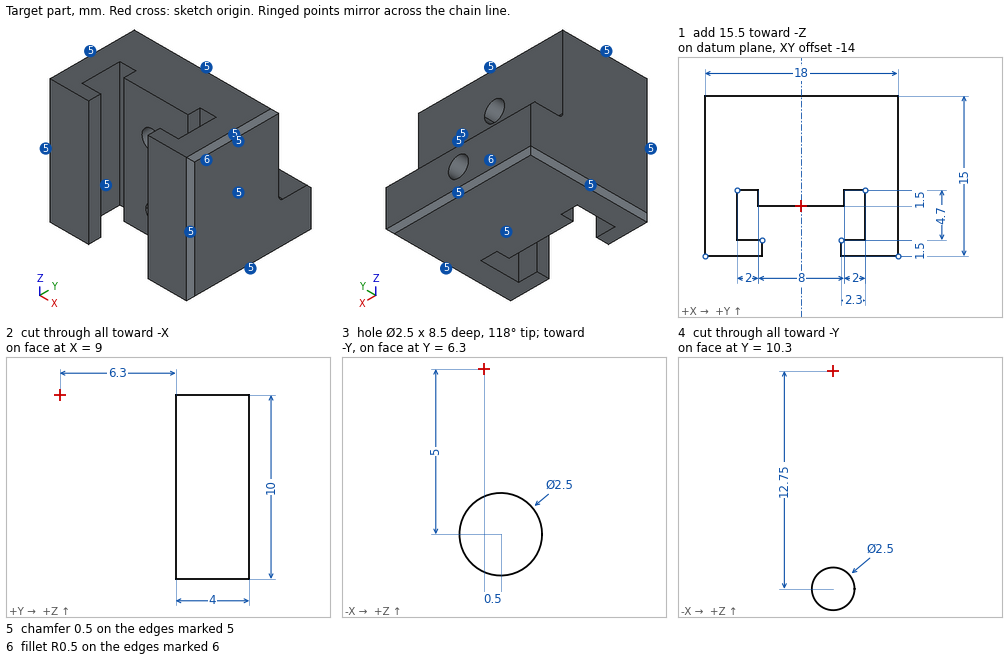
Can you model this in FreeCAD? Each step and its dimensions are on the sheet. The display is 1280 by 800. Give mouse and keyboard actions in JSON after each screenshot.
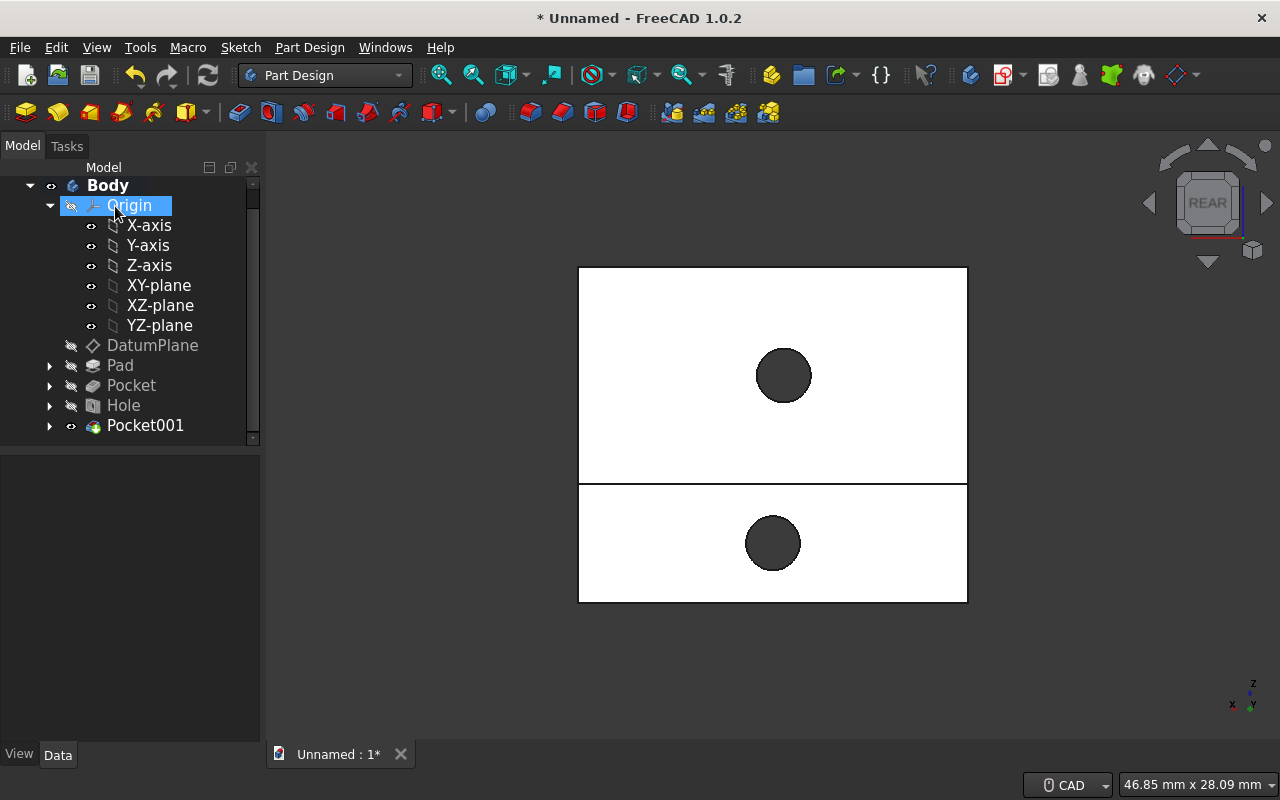
{"action": "left_click", "coordinate": [773, 602]}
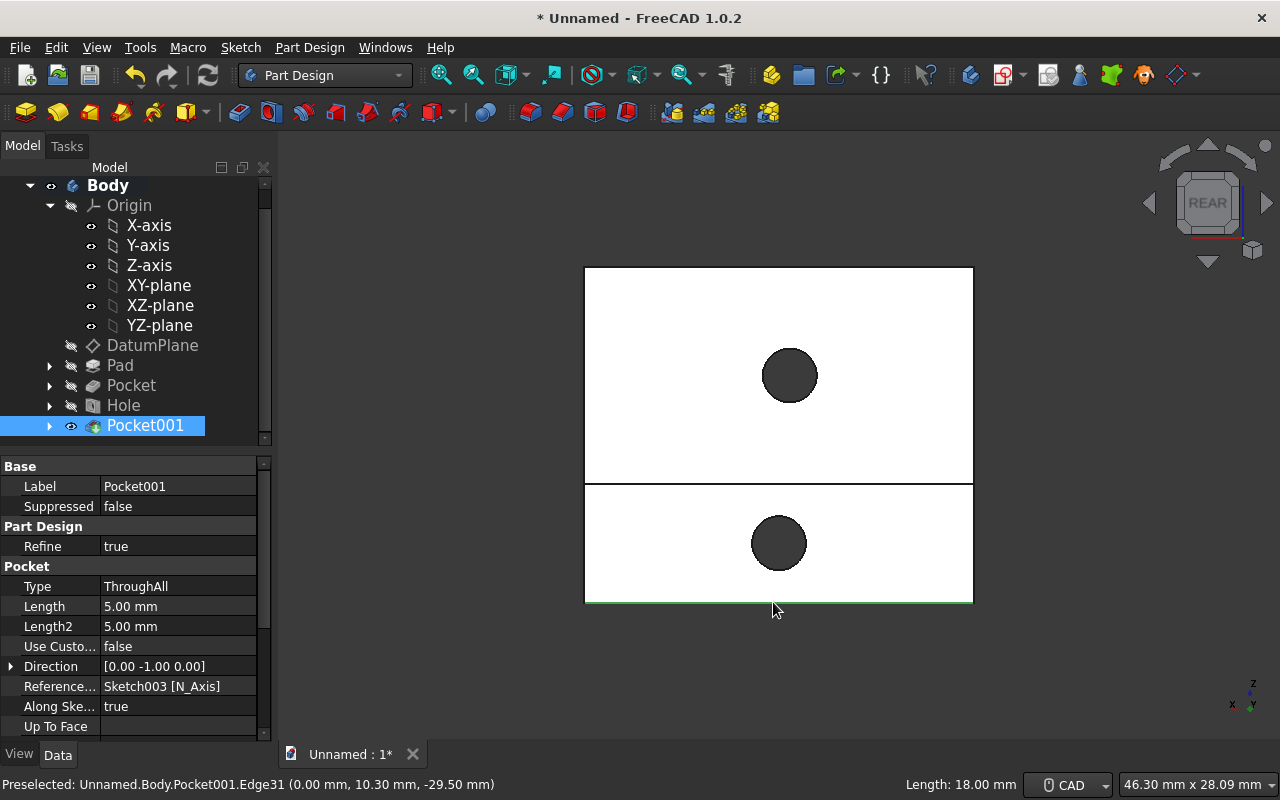
{"action": "left_click", "coordinate": [779, 266], "text": "ctrl"}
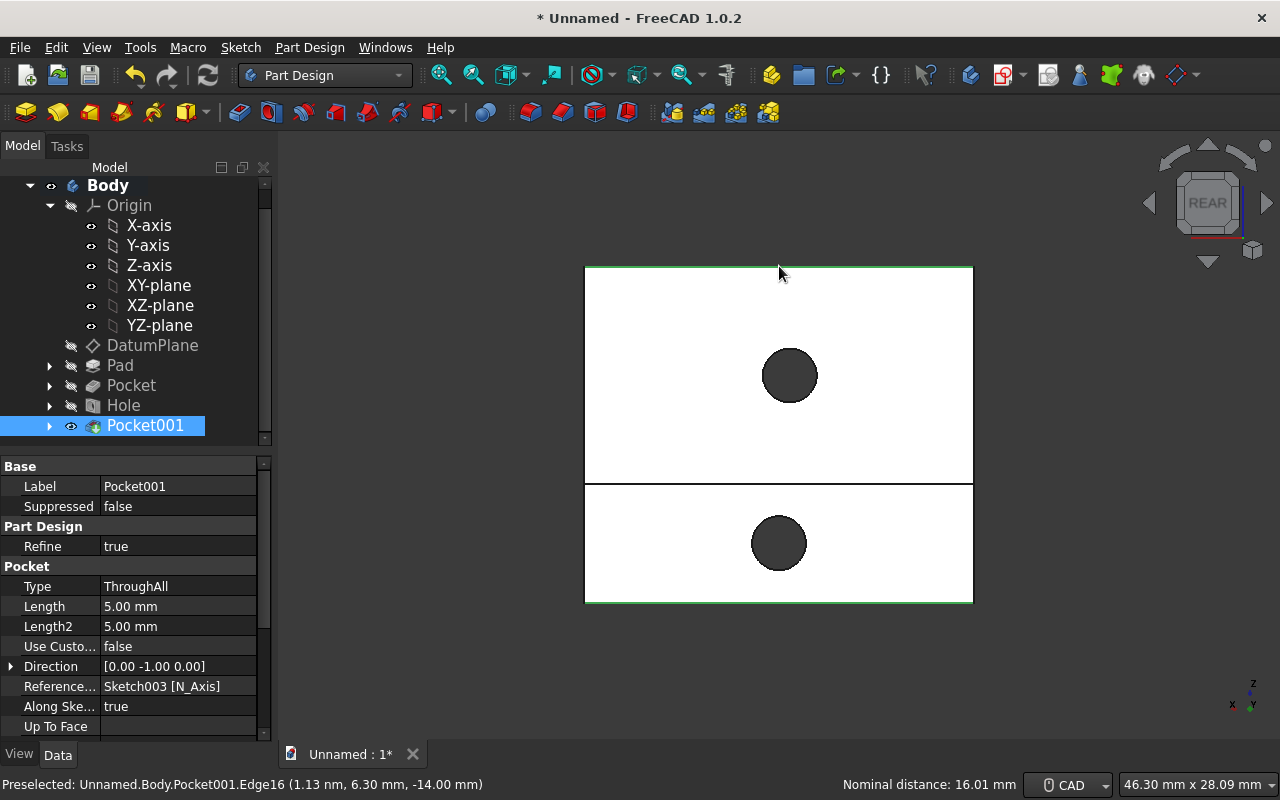
{"action": "left_click", "coordinate": [779, 483], "text": "ctrl"}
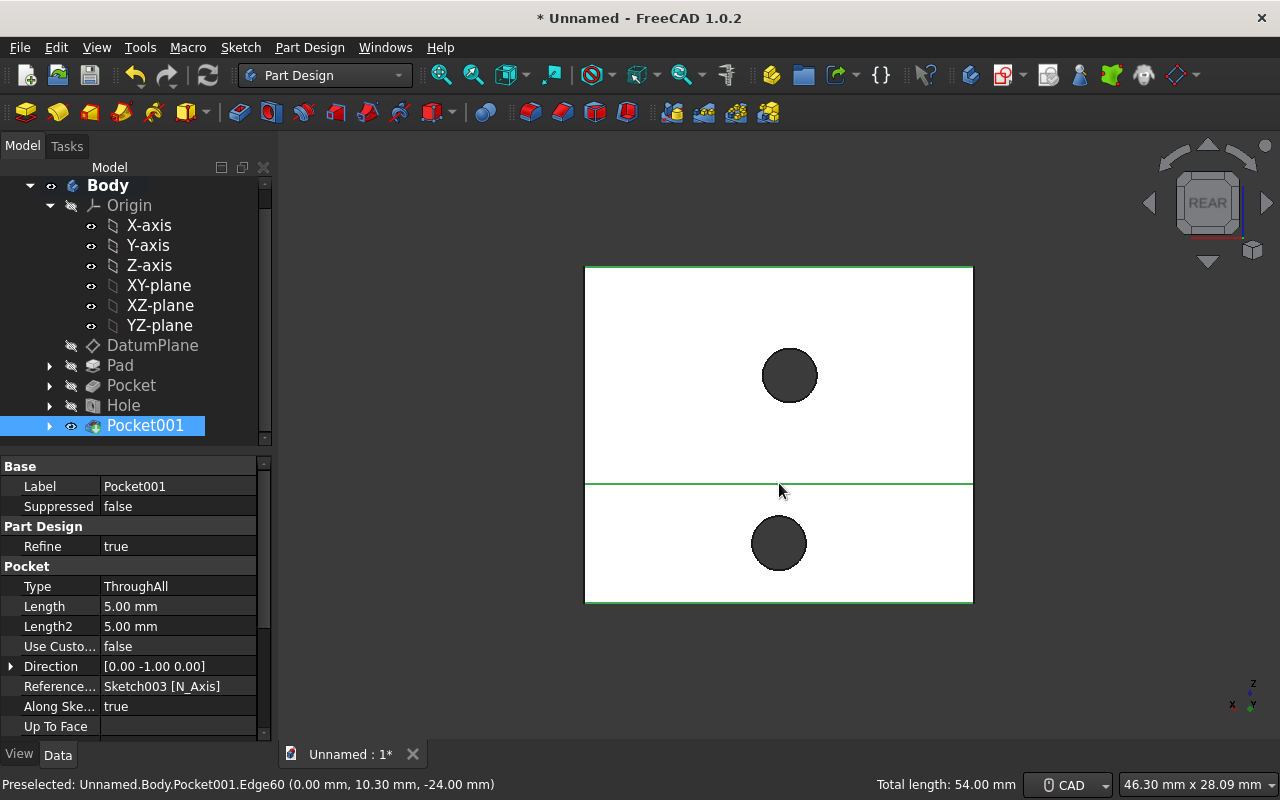
{"action": "key", "text": "0"}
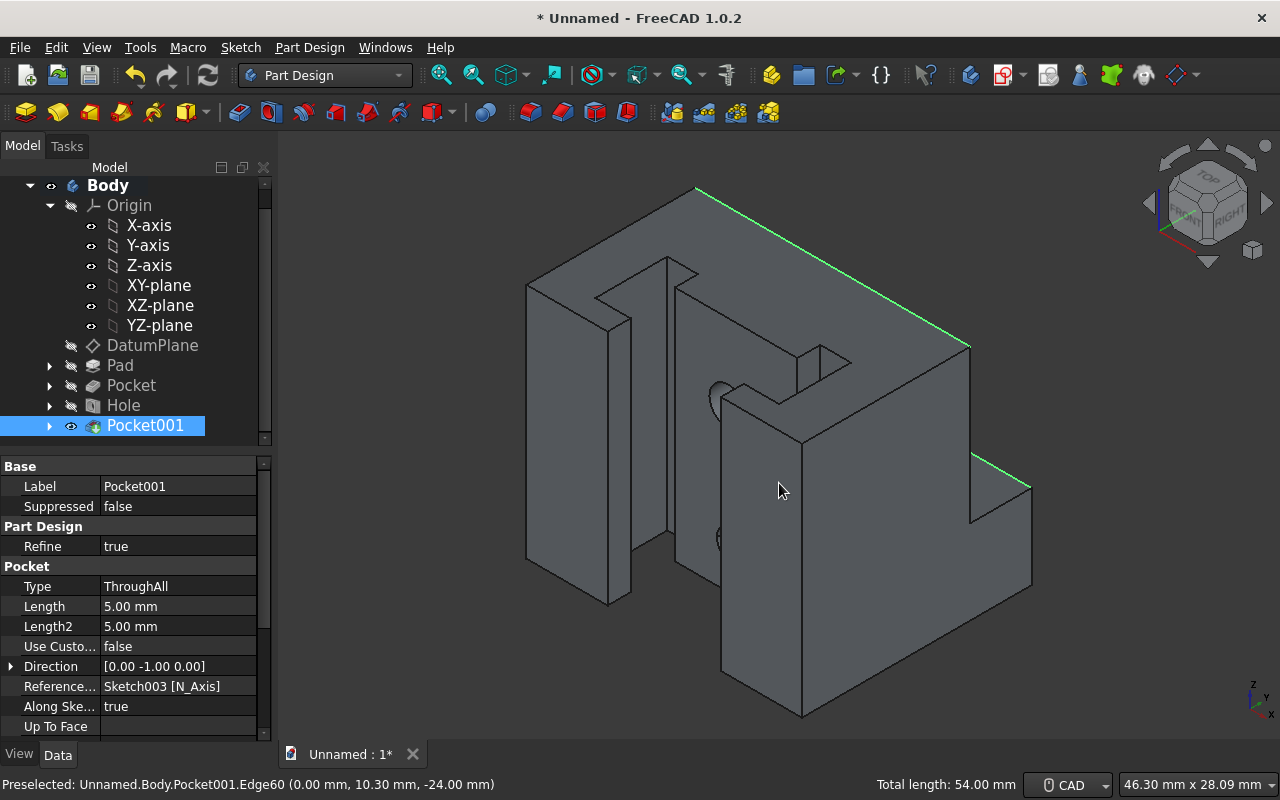
{"action": "left_click", "coordinate": [886, 394], "text": "ctrl"}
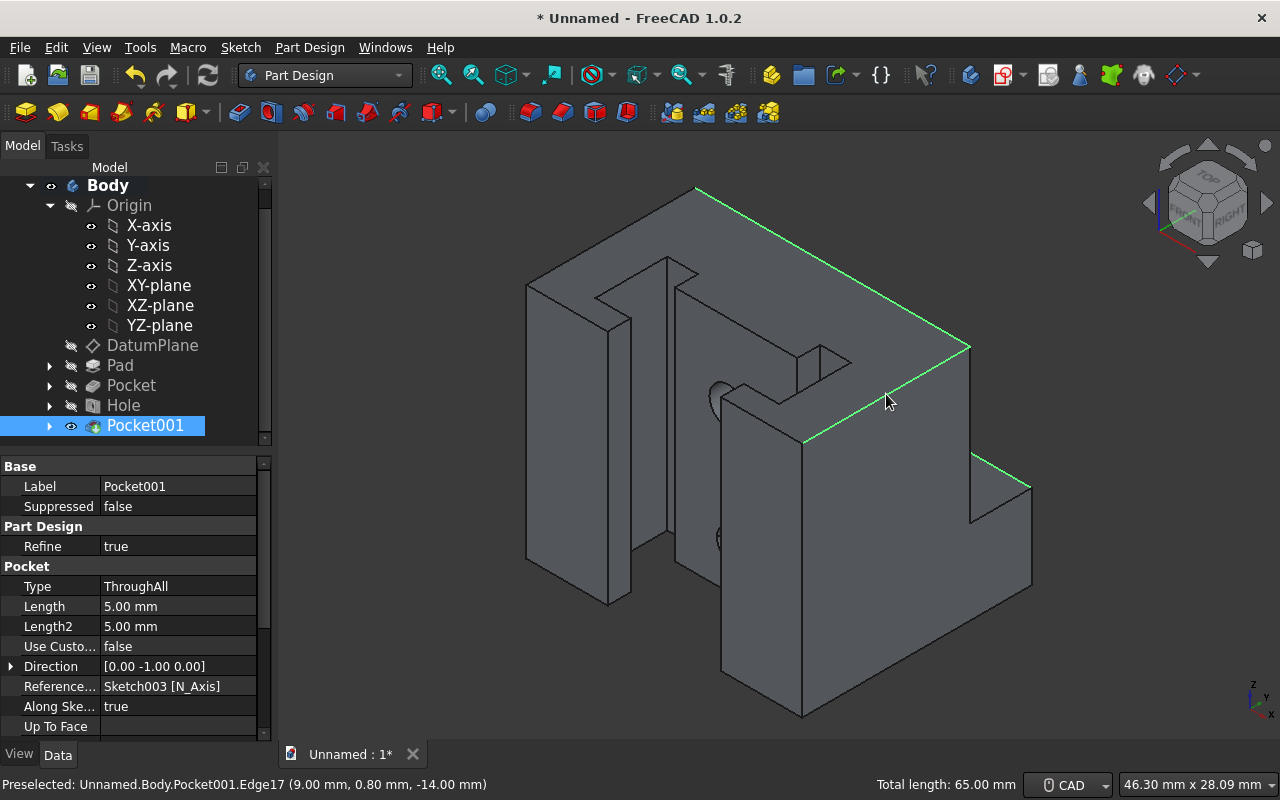
{"action": "left_click", "coordinate": [802, 580], "text": "ctrl"}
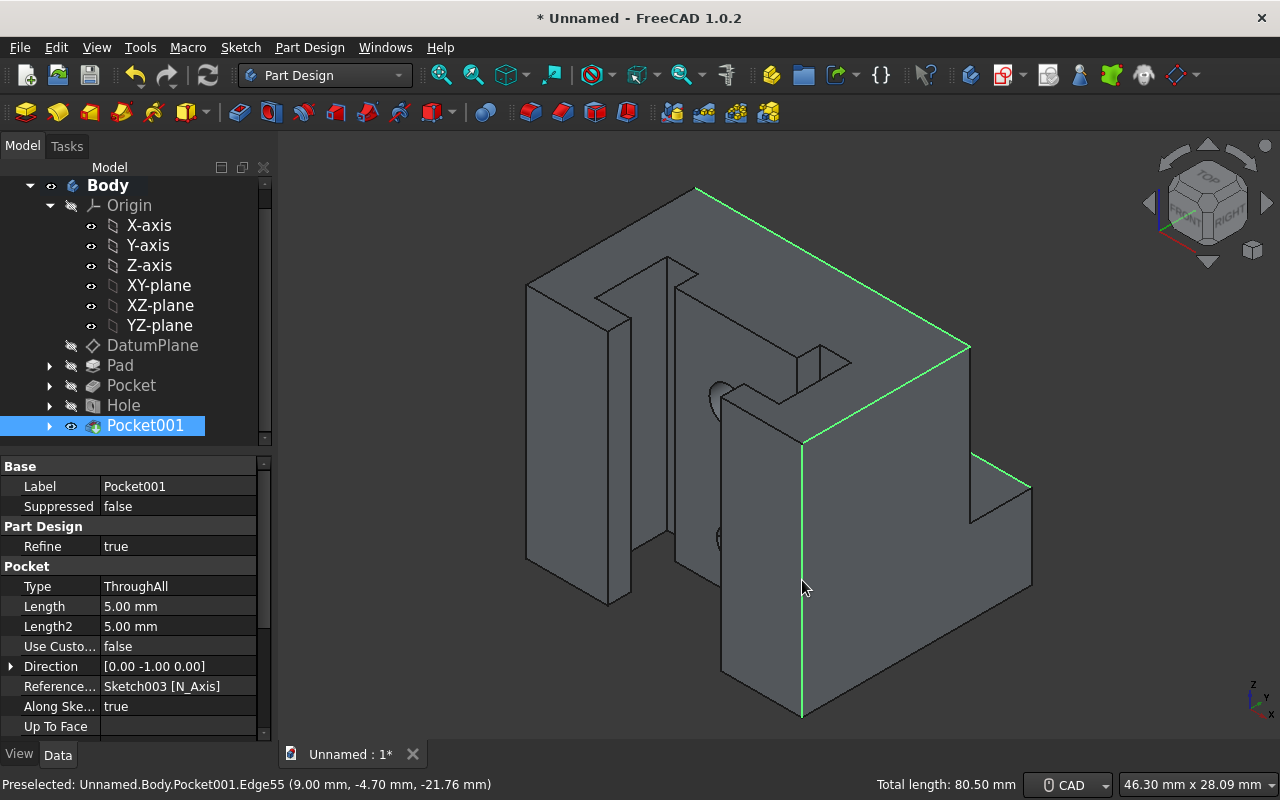
{"action": "key", "text": "2"}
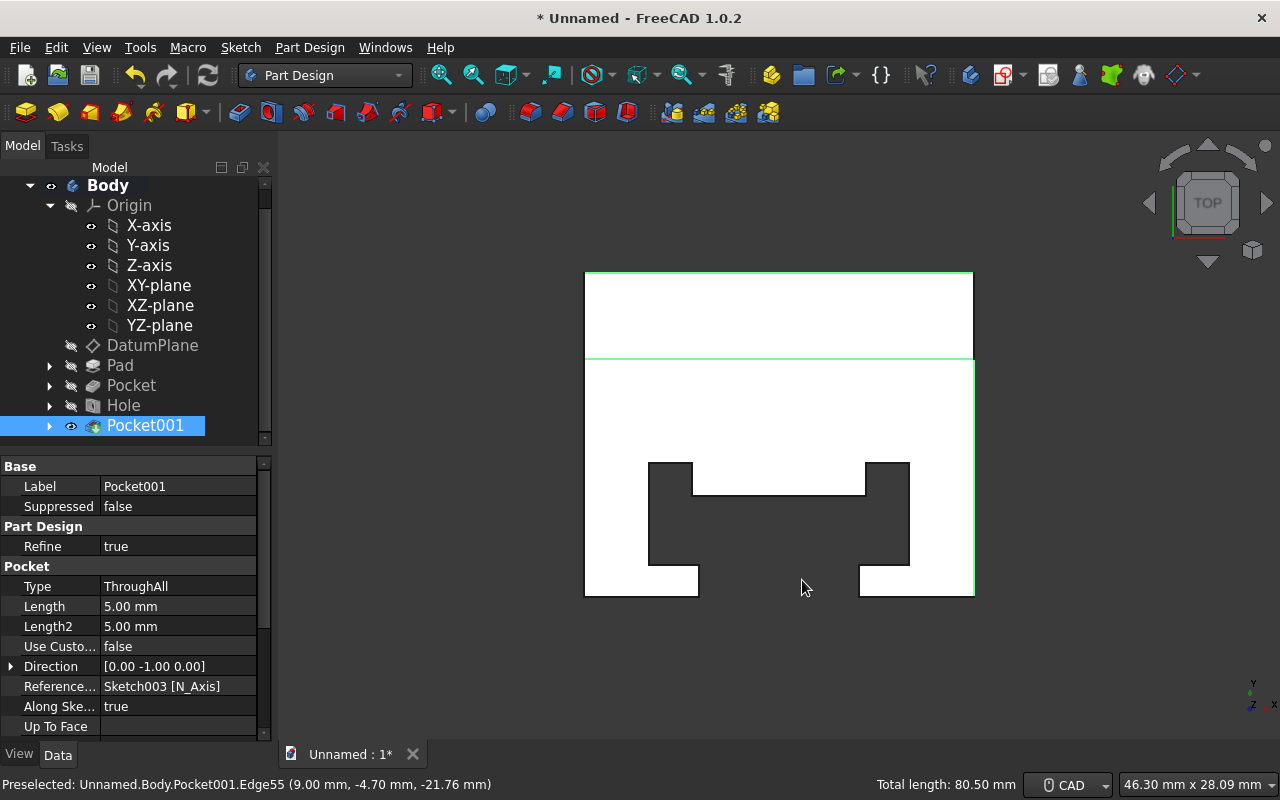
{"action": "left_click", "coordinate": [584, 477], "text": "ctrl"}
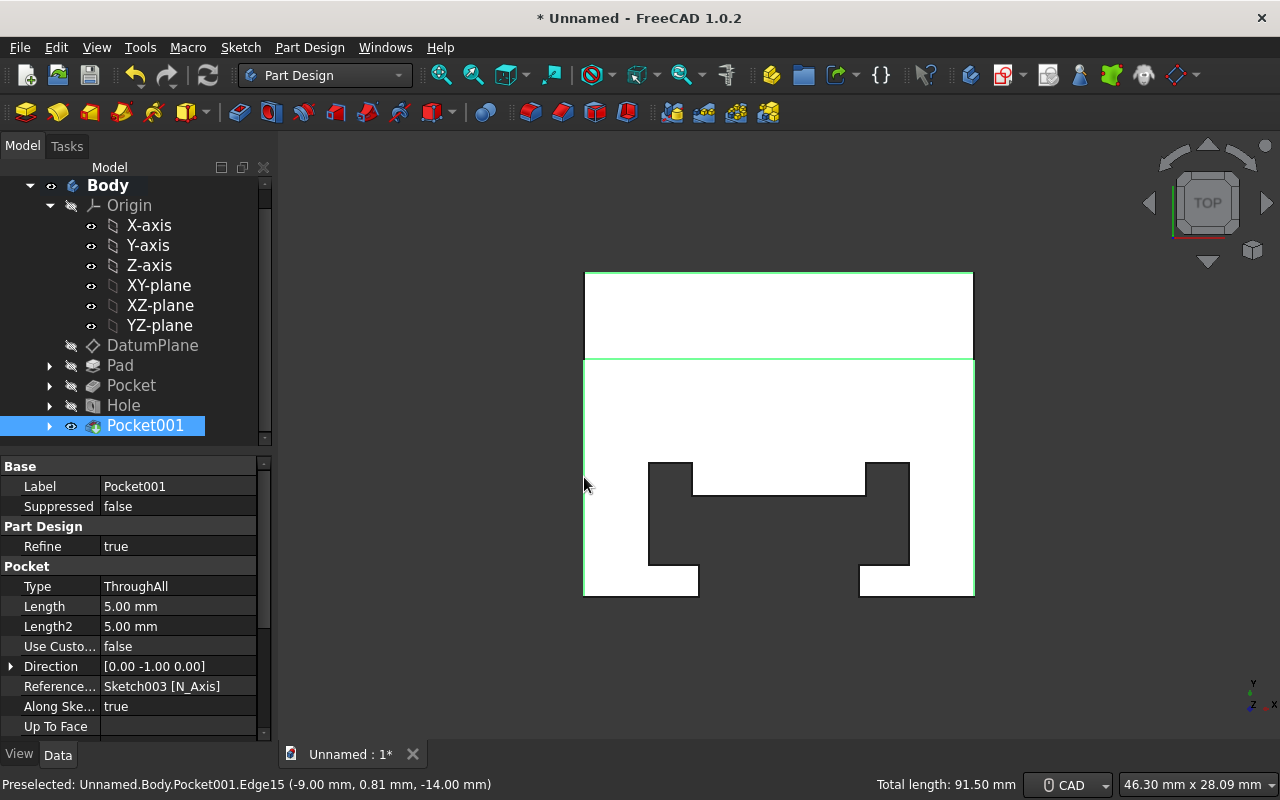
{"action": "key", "text": "1"}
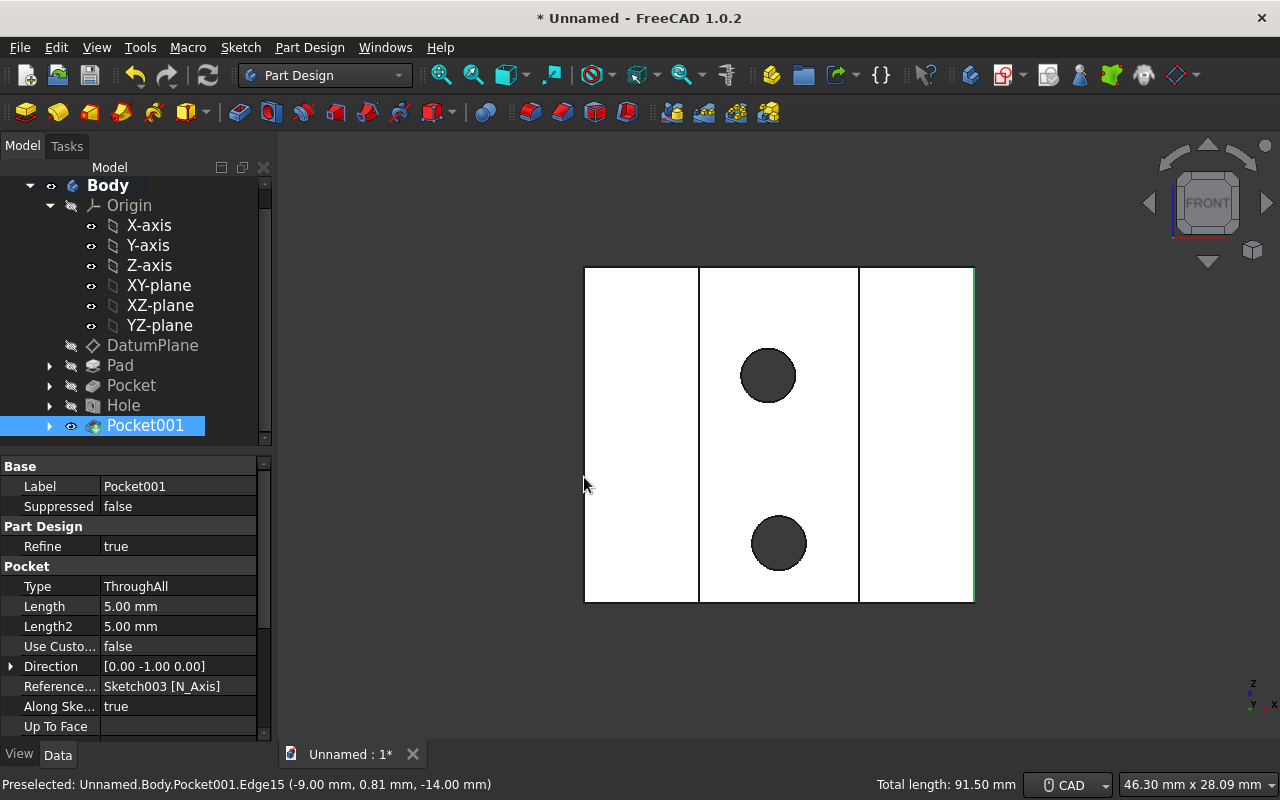
{"action": "left_click", "coordinate": [584, 434], "text": "ctrl"}